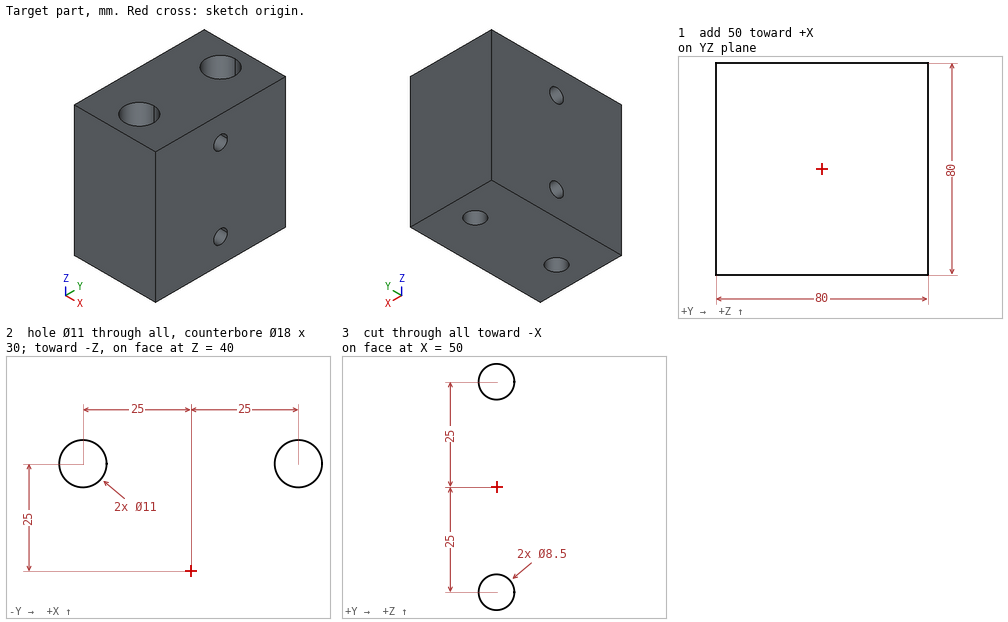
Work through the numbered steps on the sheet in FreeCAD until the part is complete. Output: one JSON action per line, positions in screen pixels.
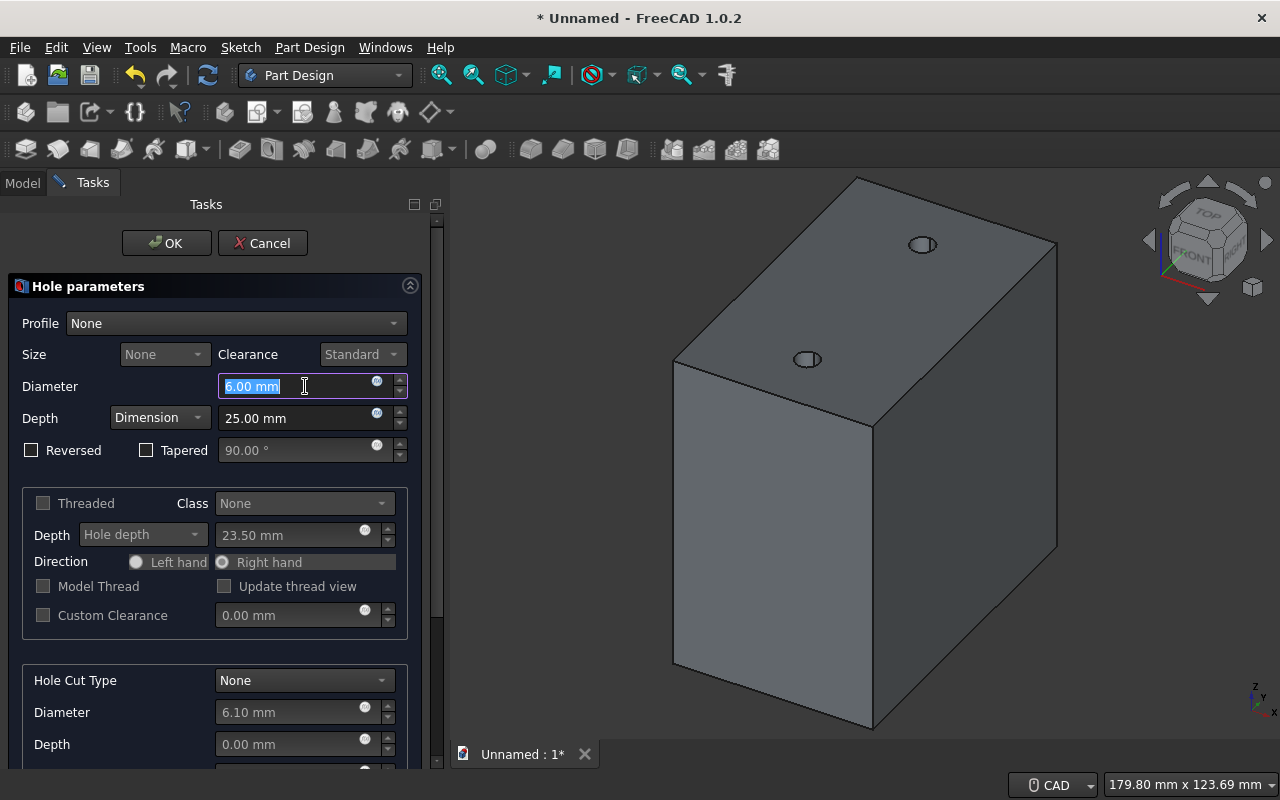
{"action": "type", "text": "11"}
{"action": "key", "text": "Tab"}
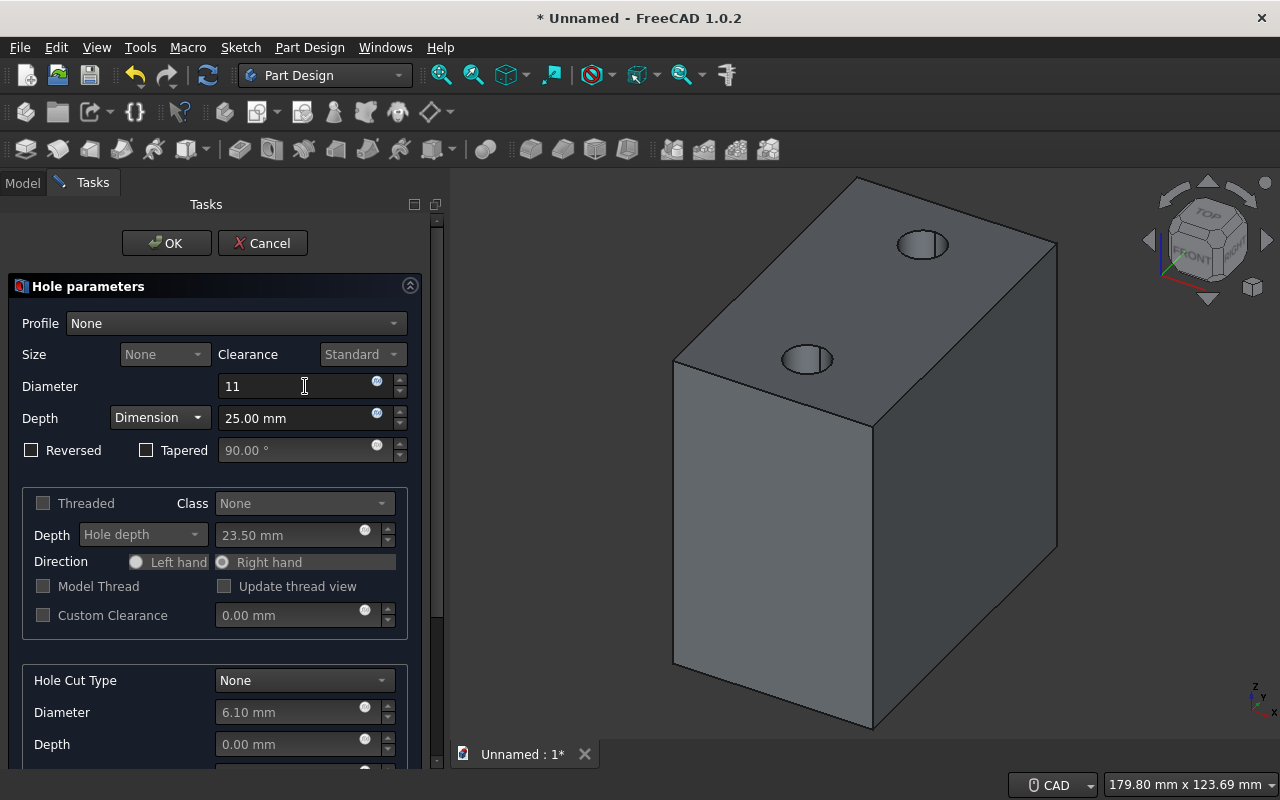
{"action": "left_click", "coordinate": [161, 418]}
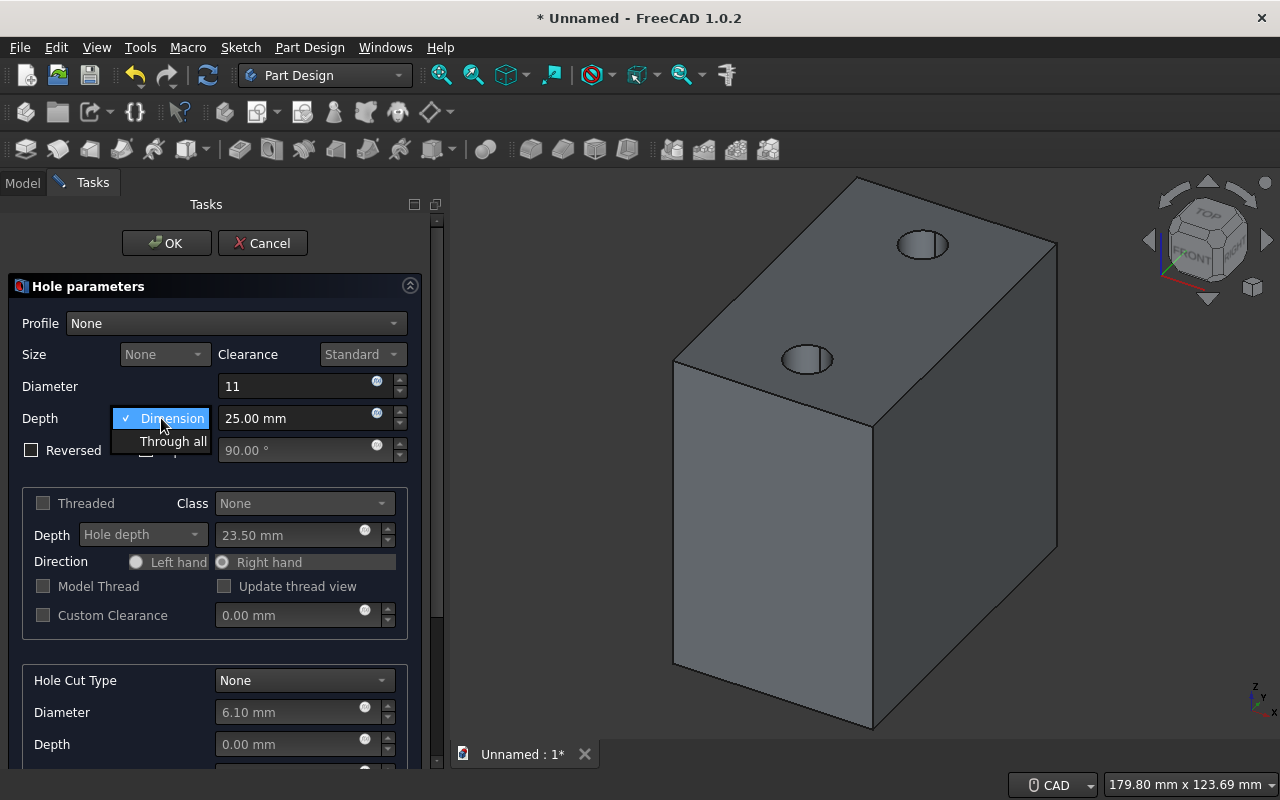
{"action": "left_click", "coordinate": [160, 442]}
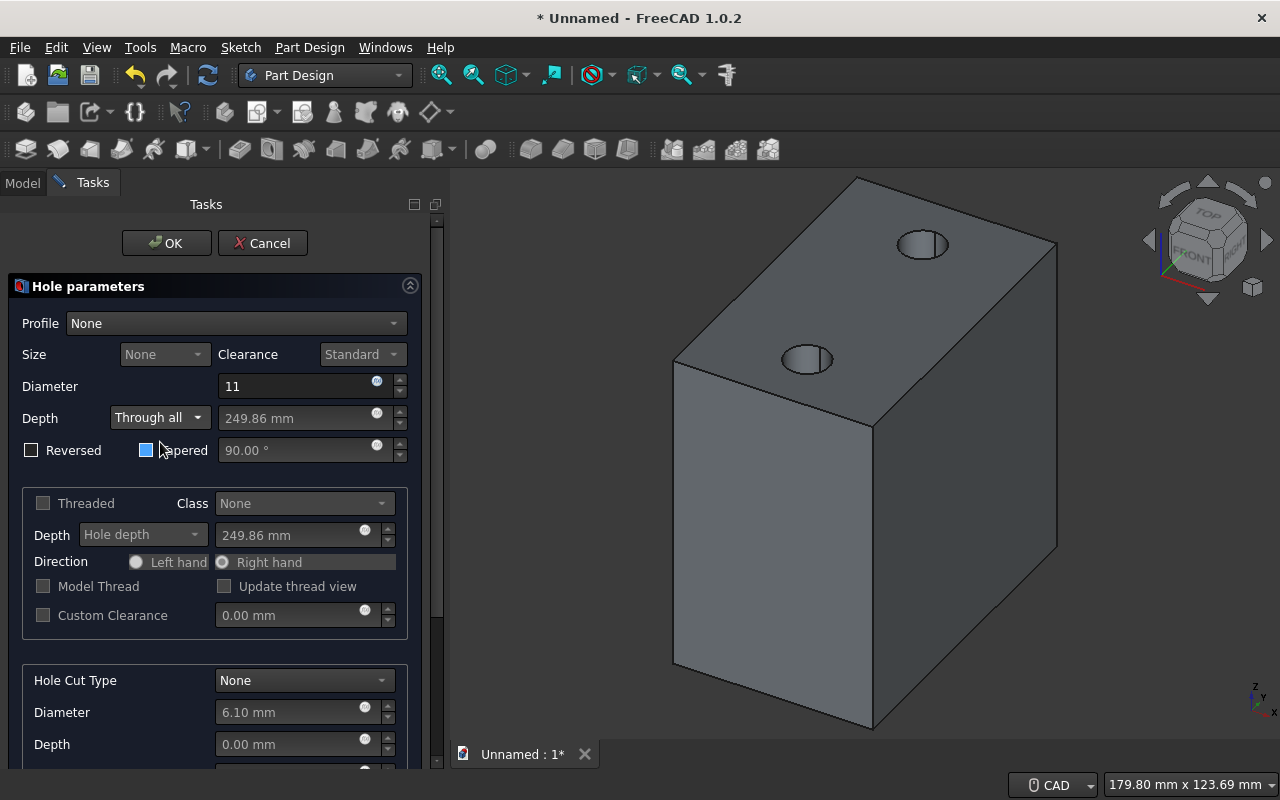
{"action": "left_click", "coordinate": [306, 680]}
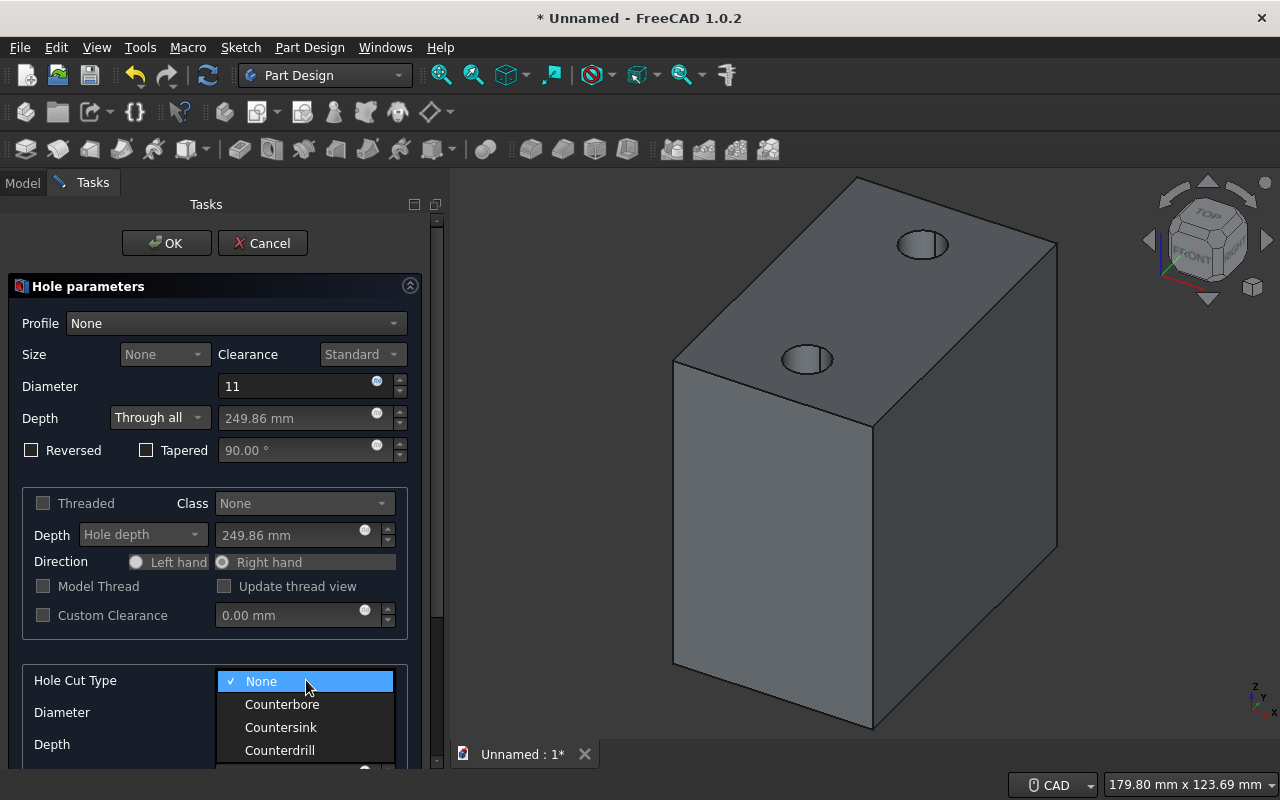
{"action": "left_click", "coordinate": [304, 704]}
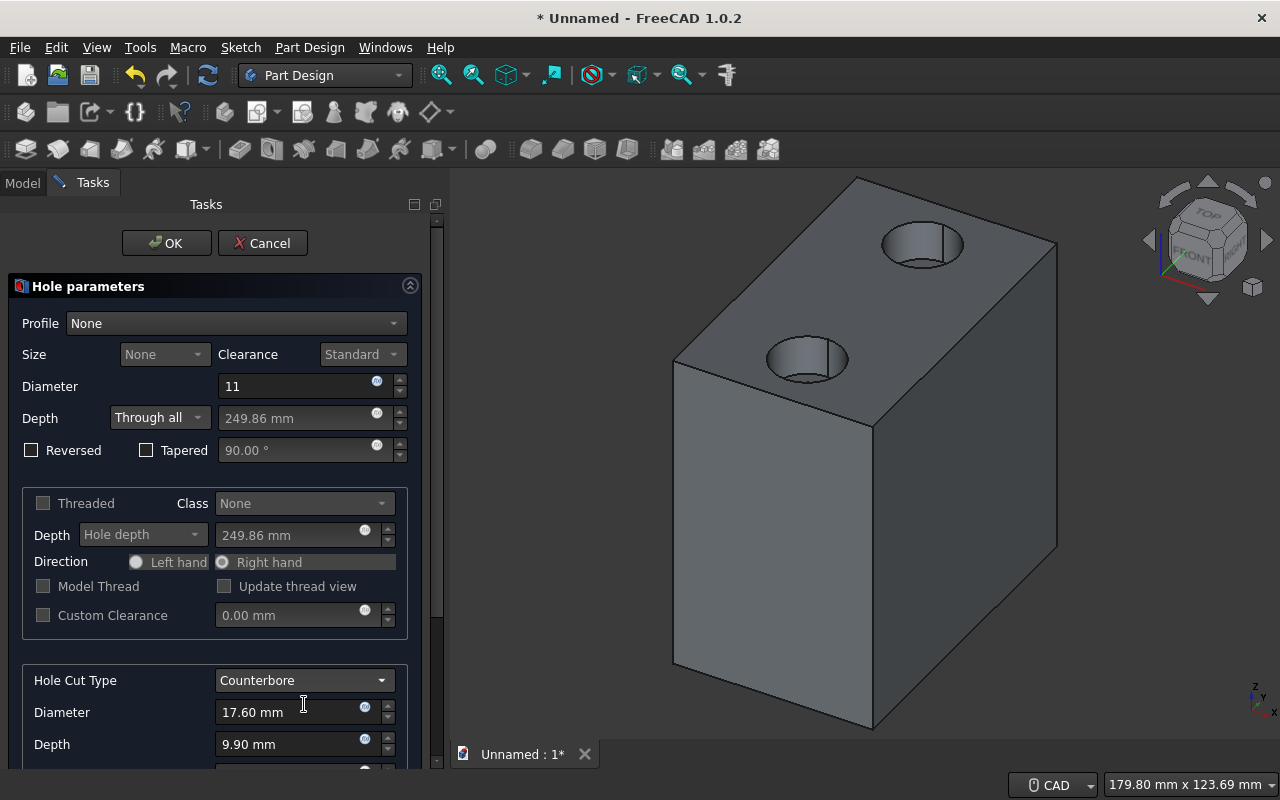
{"action": "triple_click", "coordinate": [298, 712]}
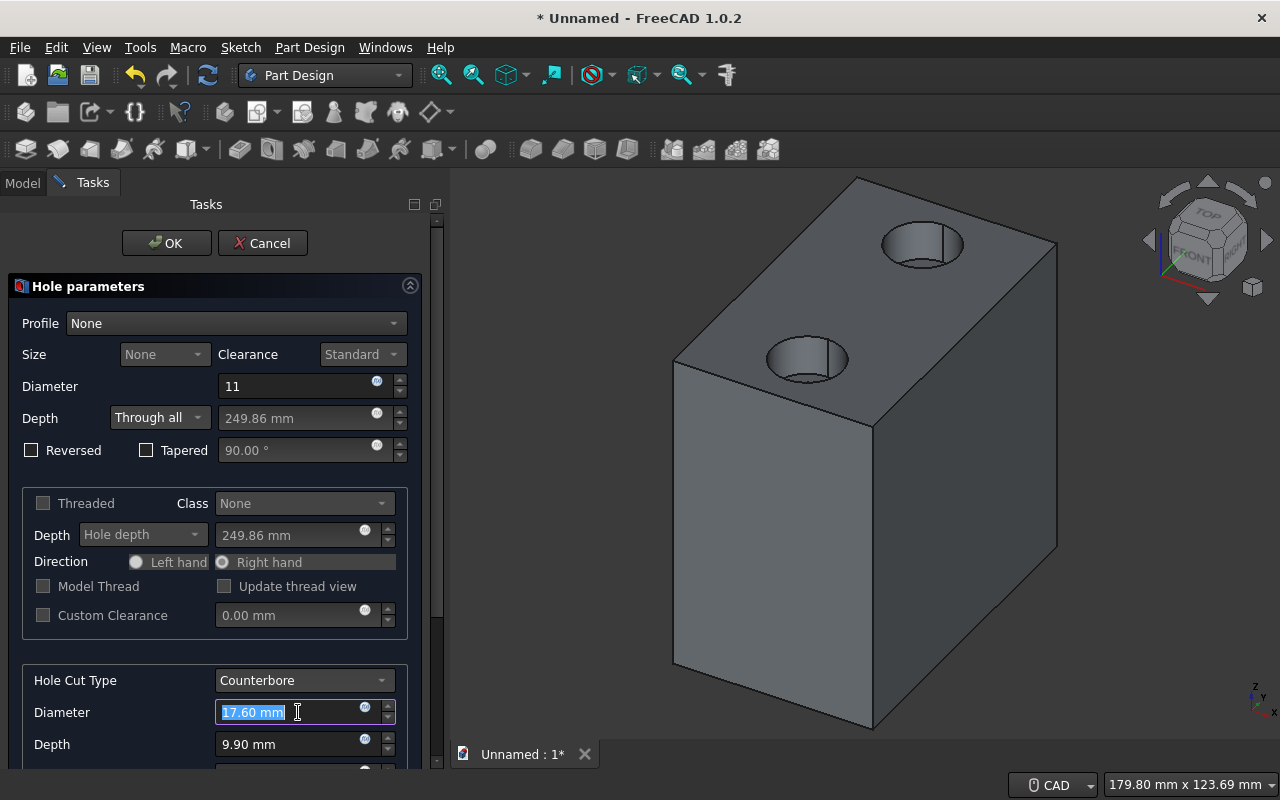
{"action": "type", "text": "18"}
{"action": "key", "text": "Tab"}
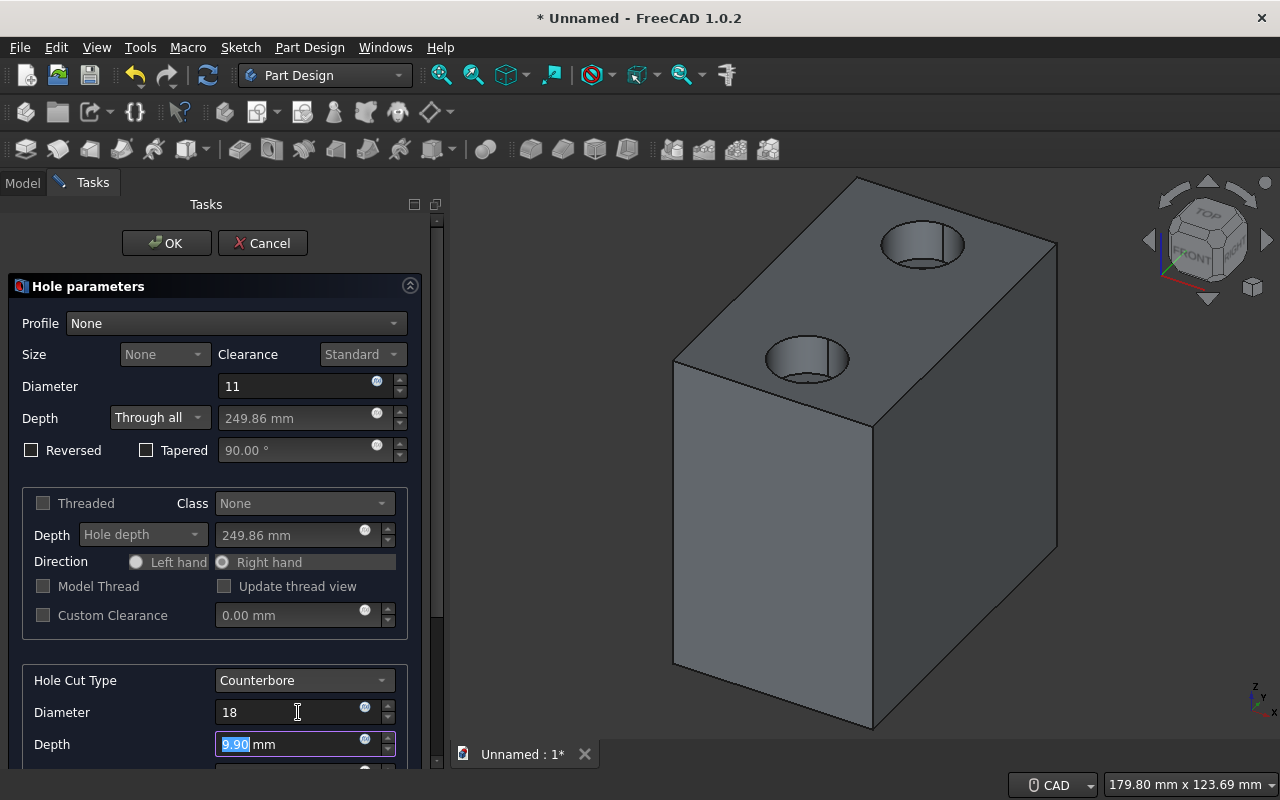
{"action": "type", "text": "30"}
{"action": "key", "text": "Tab"}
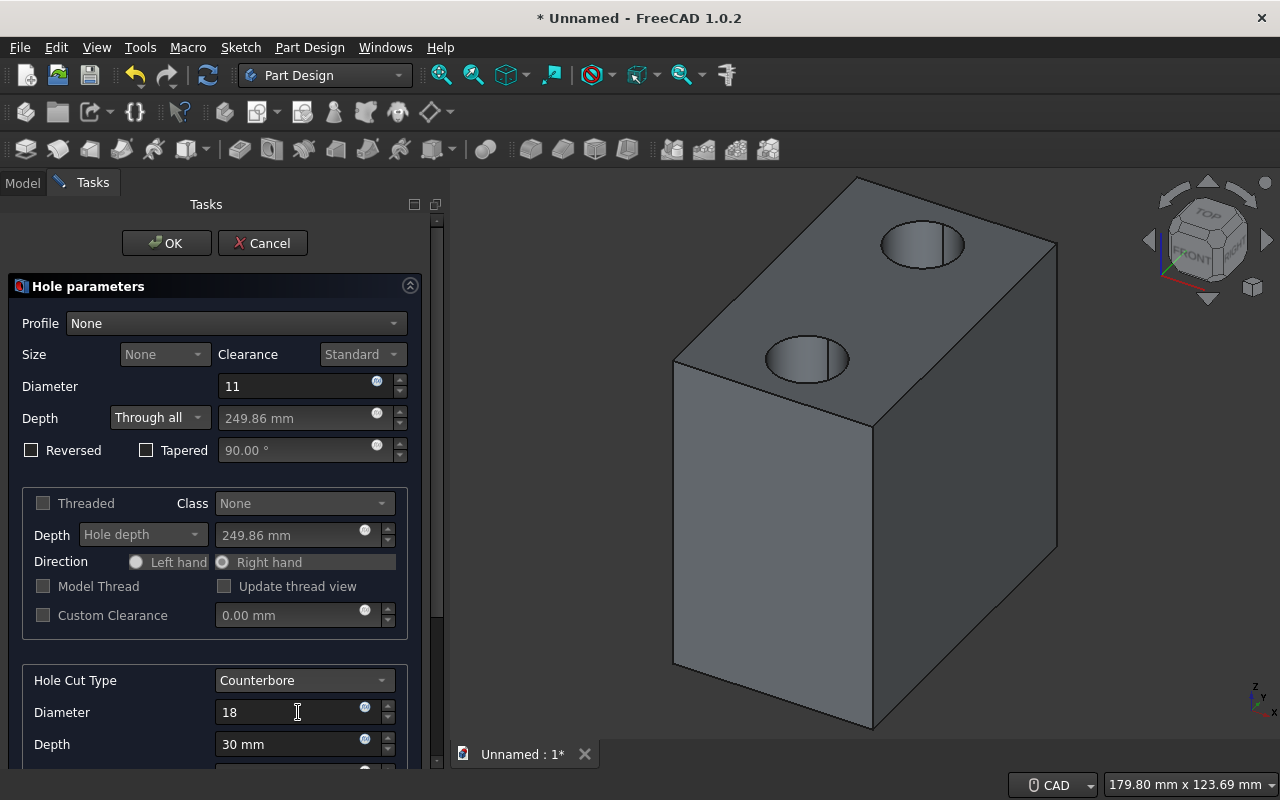
{"action": "left_click", "coordinate": [167, 243]}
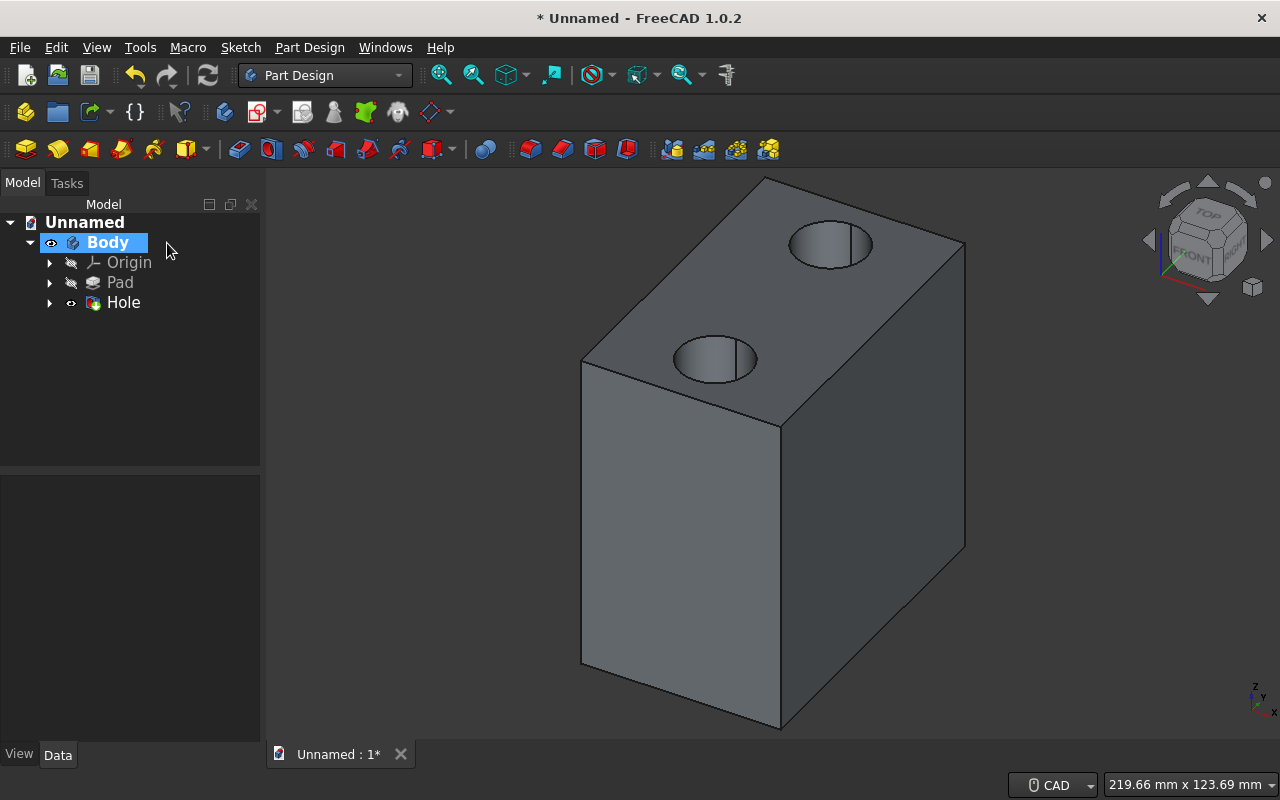
{"action": "left_click", "coordinate": [873, 486]}